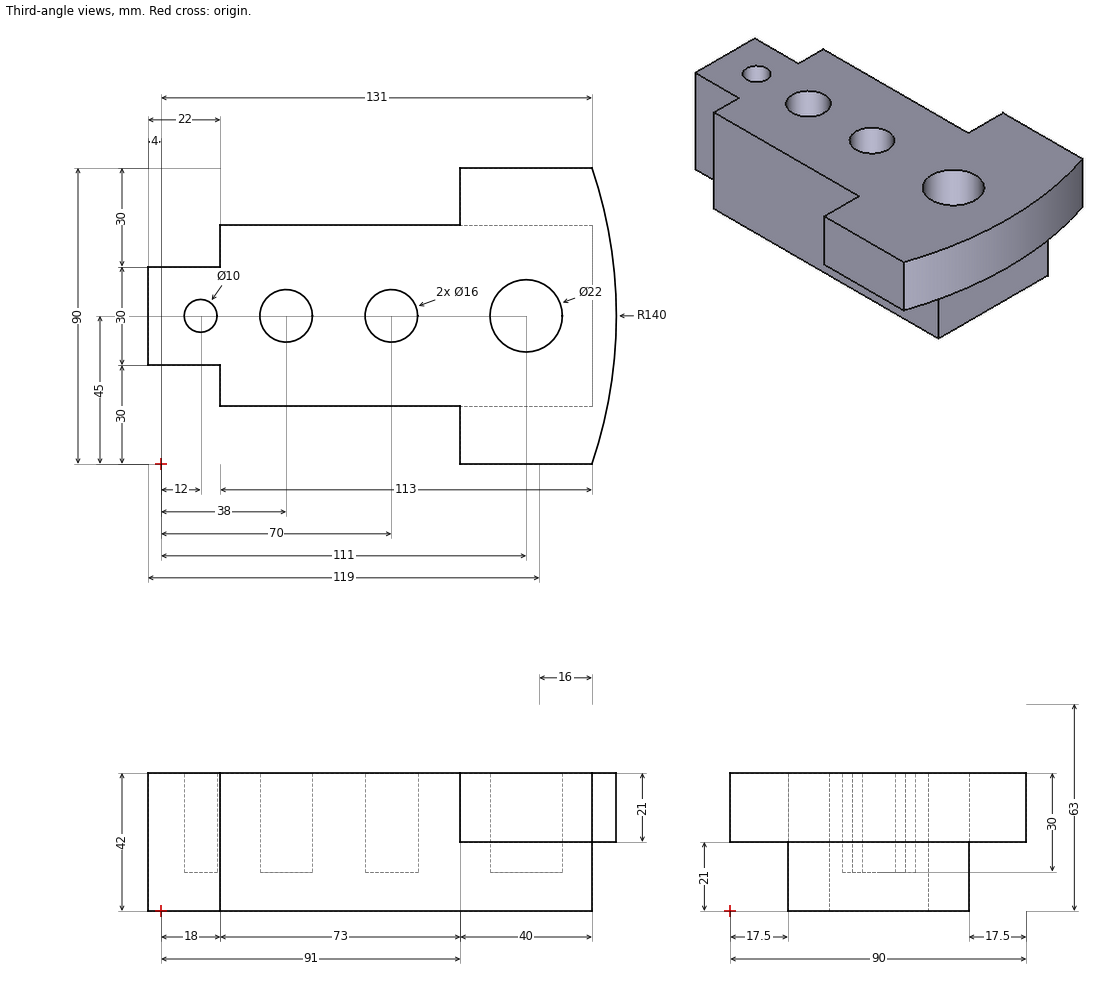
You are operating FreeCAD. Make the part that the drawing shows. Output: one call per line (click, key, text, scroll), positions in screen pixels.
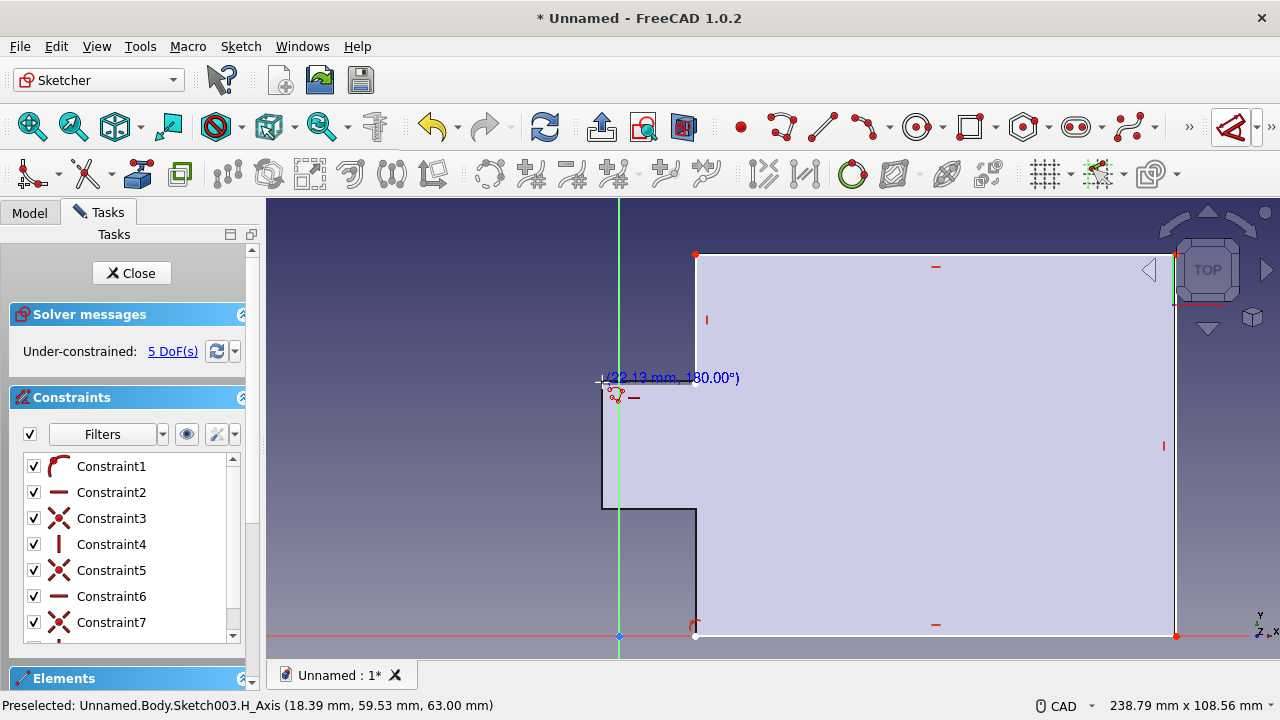
click(602, 382)
click(602, 509)
click(696, 509)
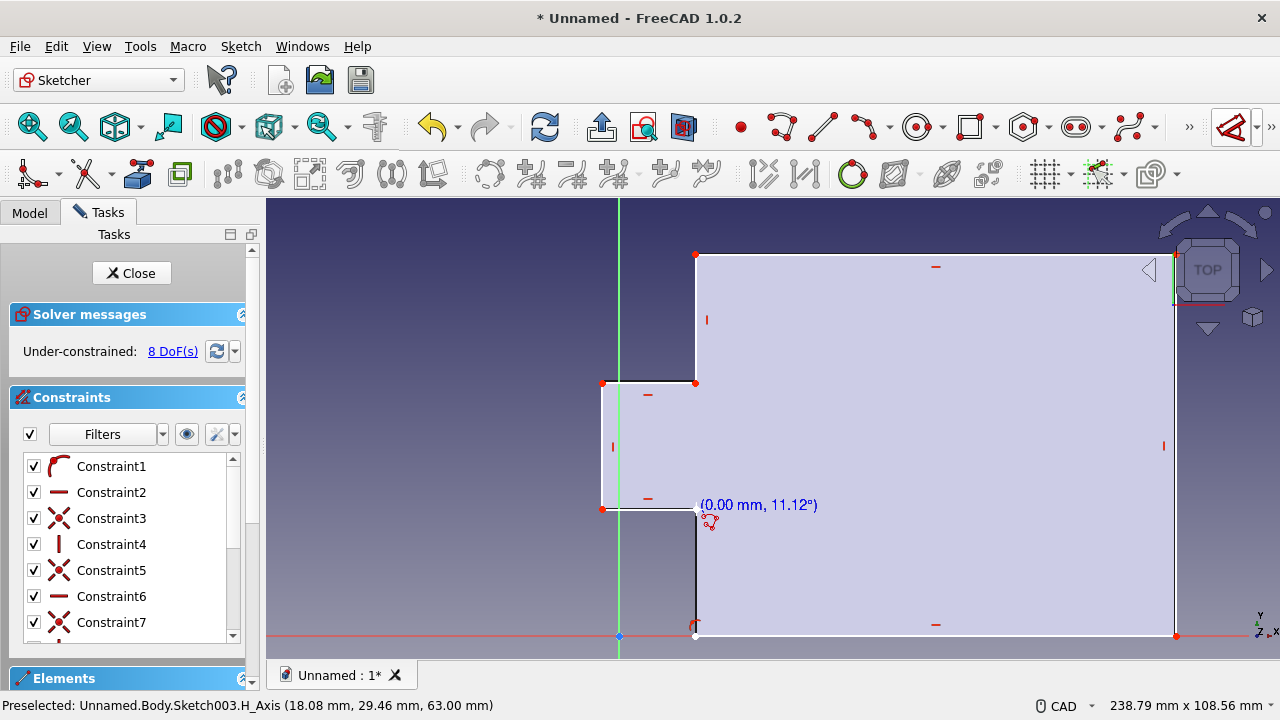
scroll(294, 354, down, 1)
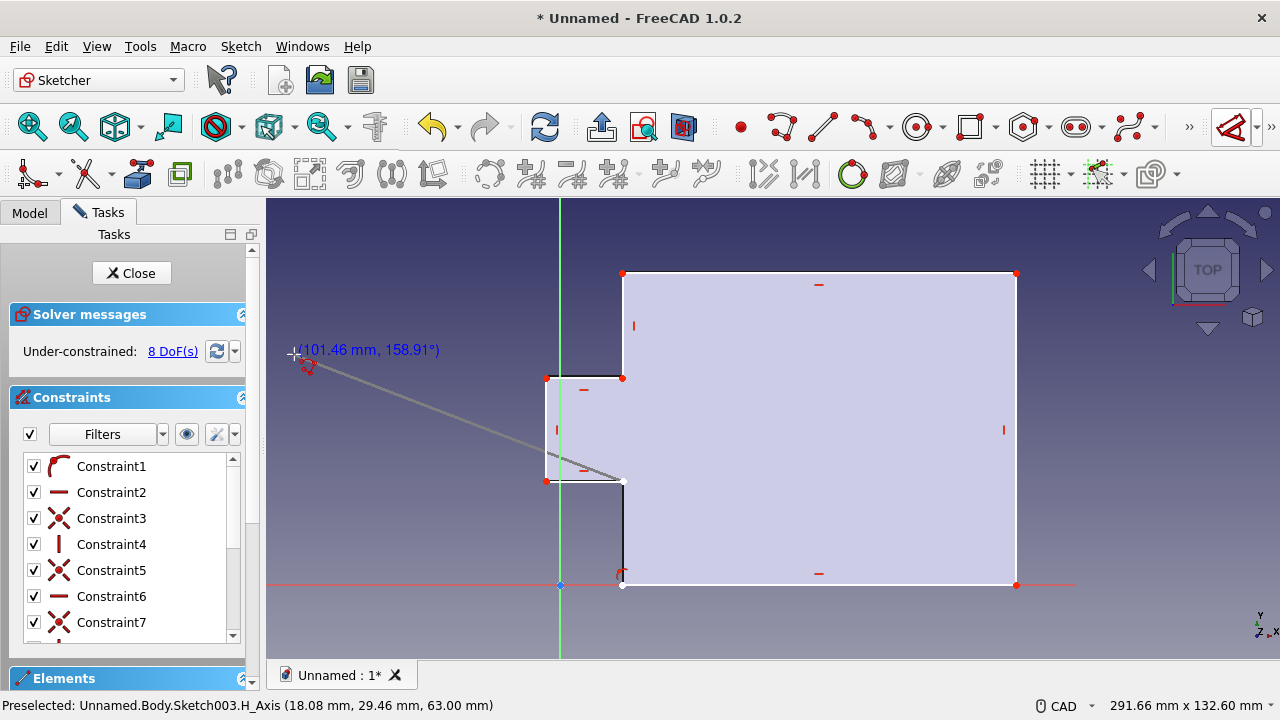
click(623, 585)
key(Escape)
key(Escape)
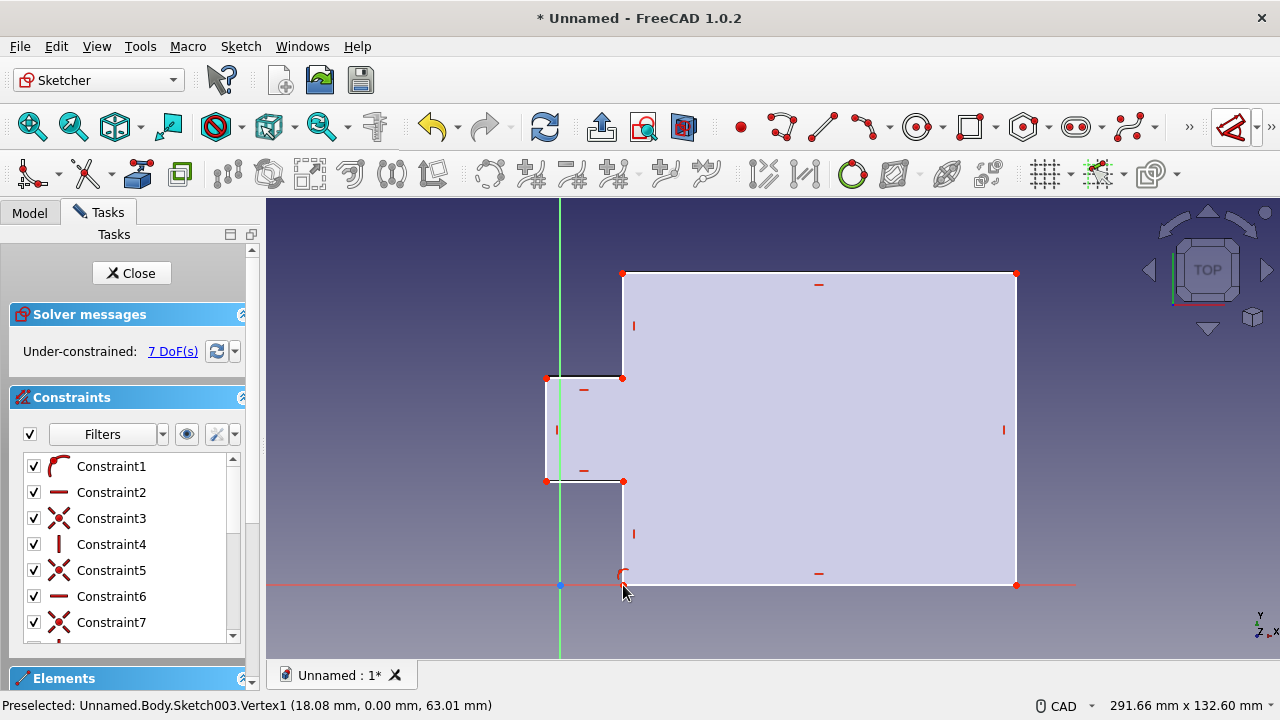
click(1016, 491)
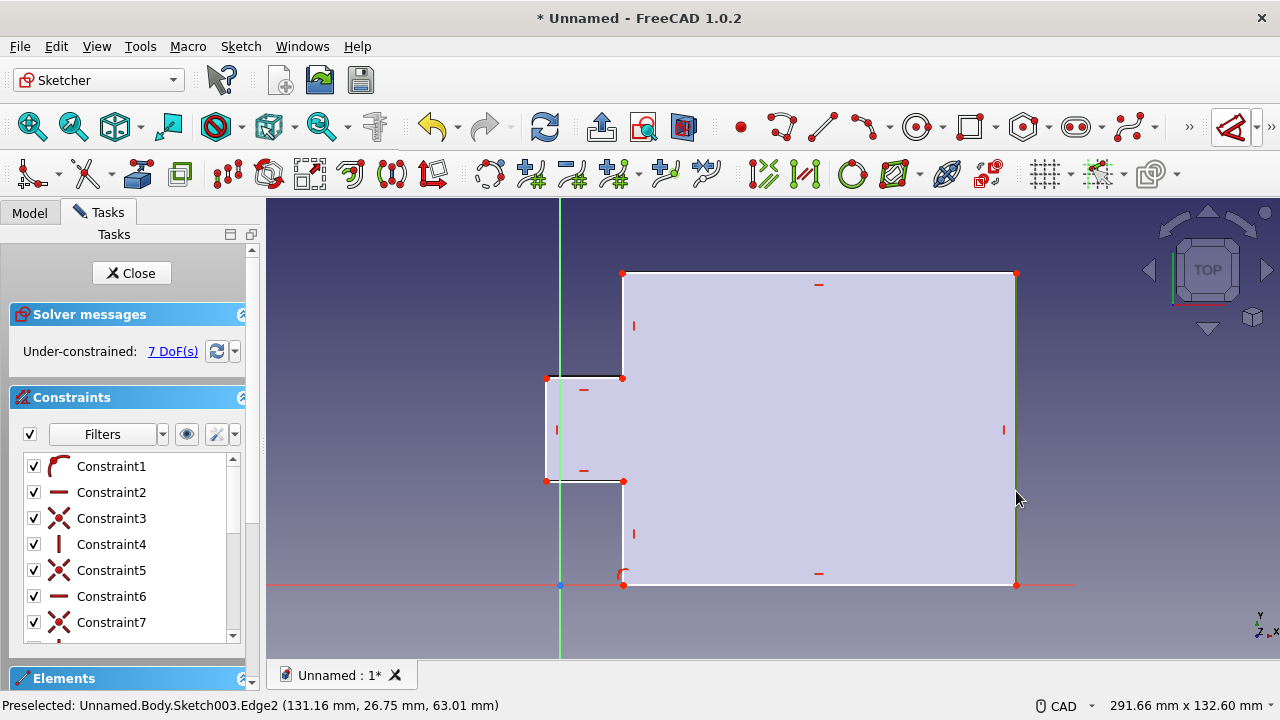
key(i)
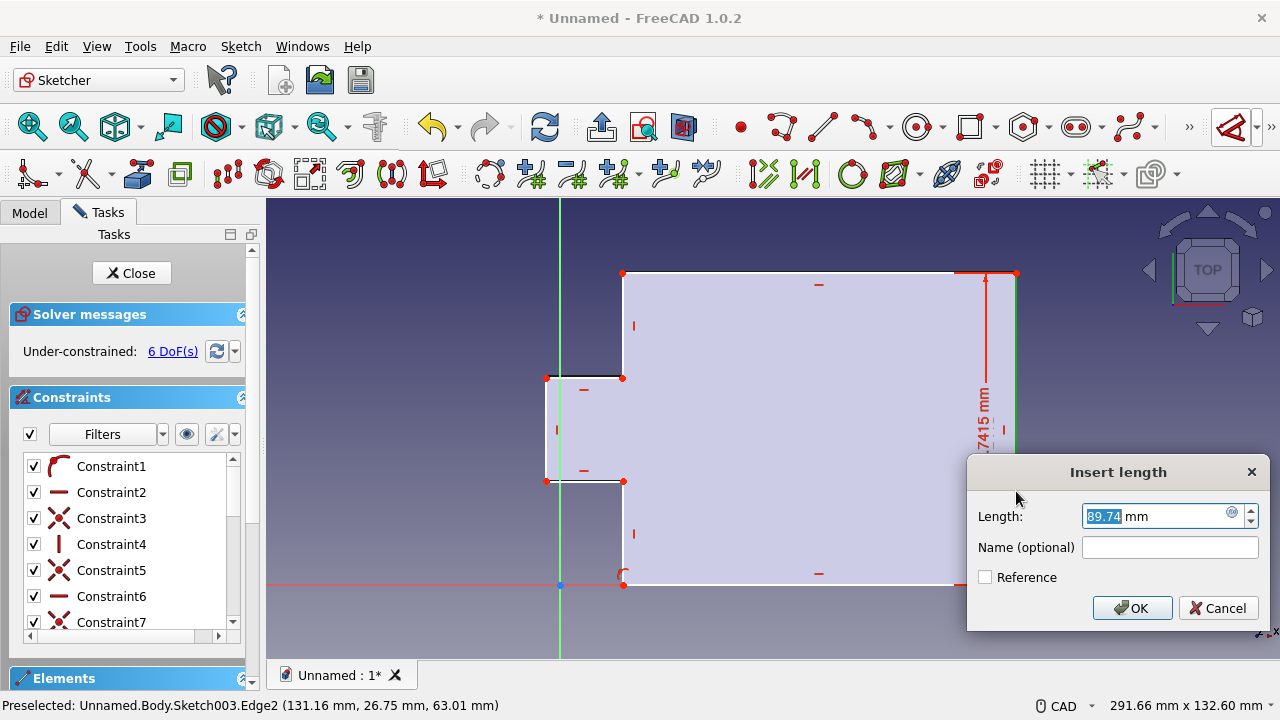
text(90)
key(Return)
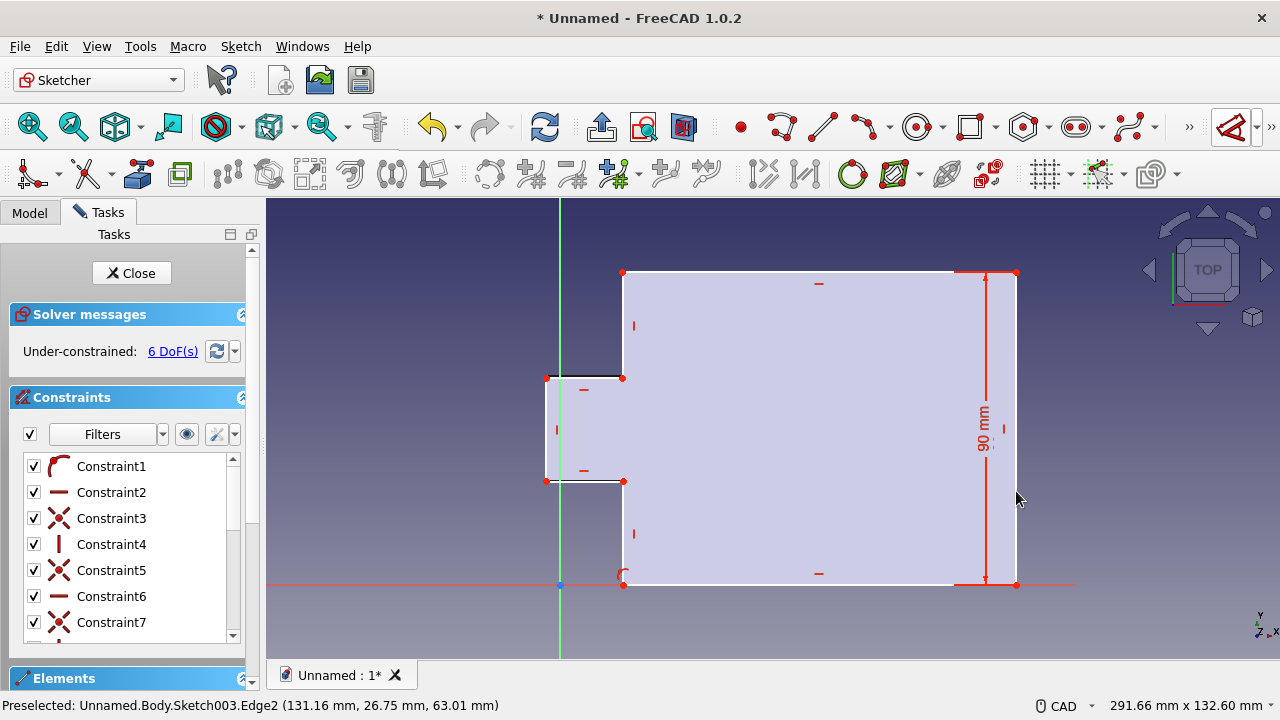
click(623, 304)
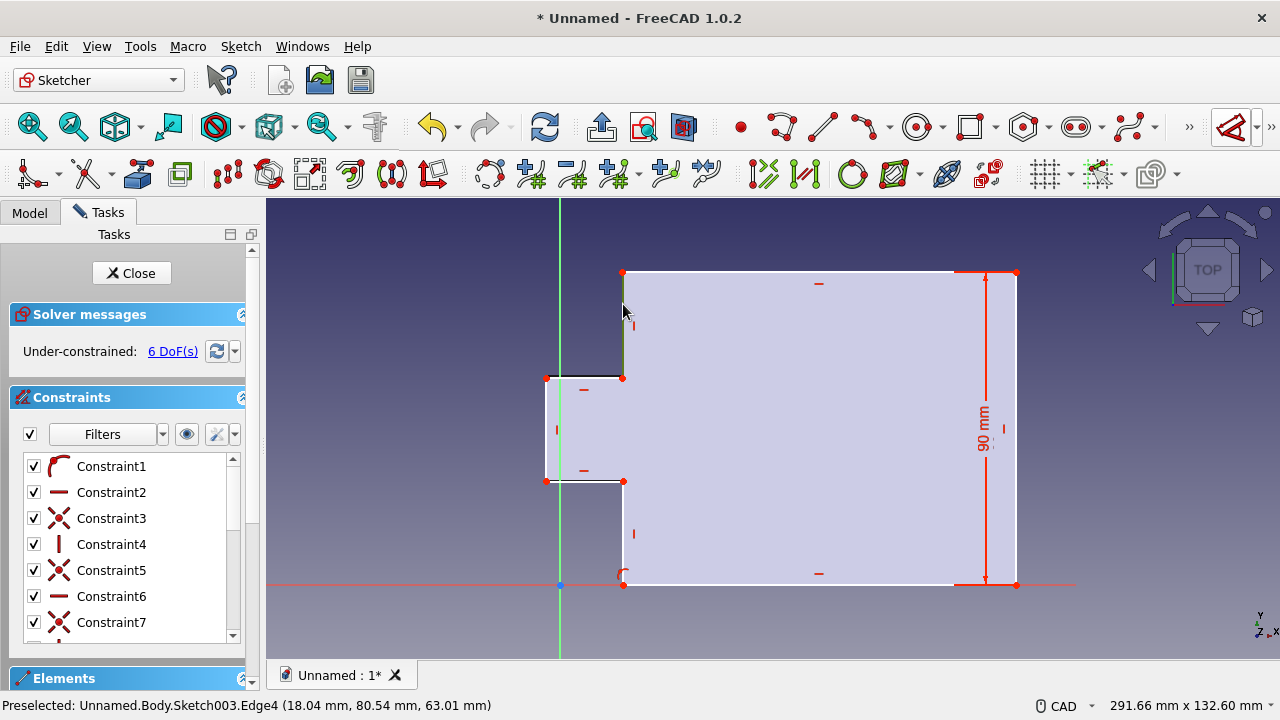
click(1256, 128)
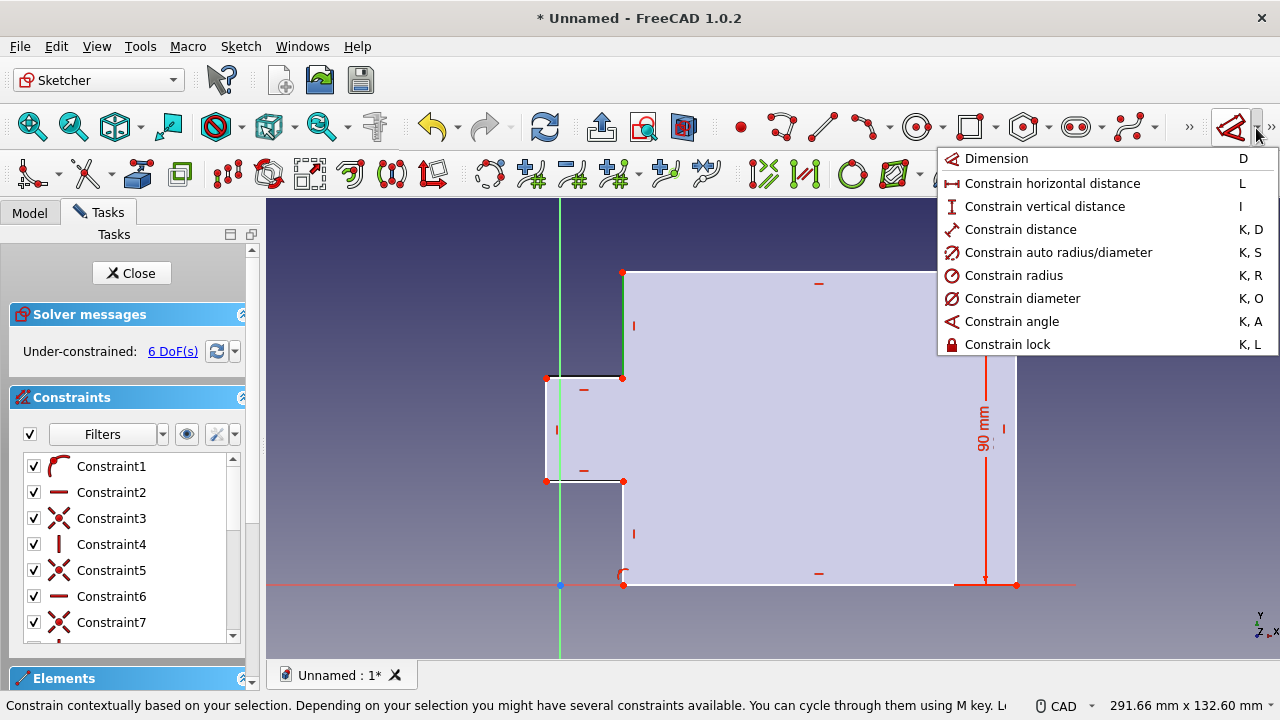
click(1108, 206)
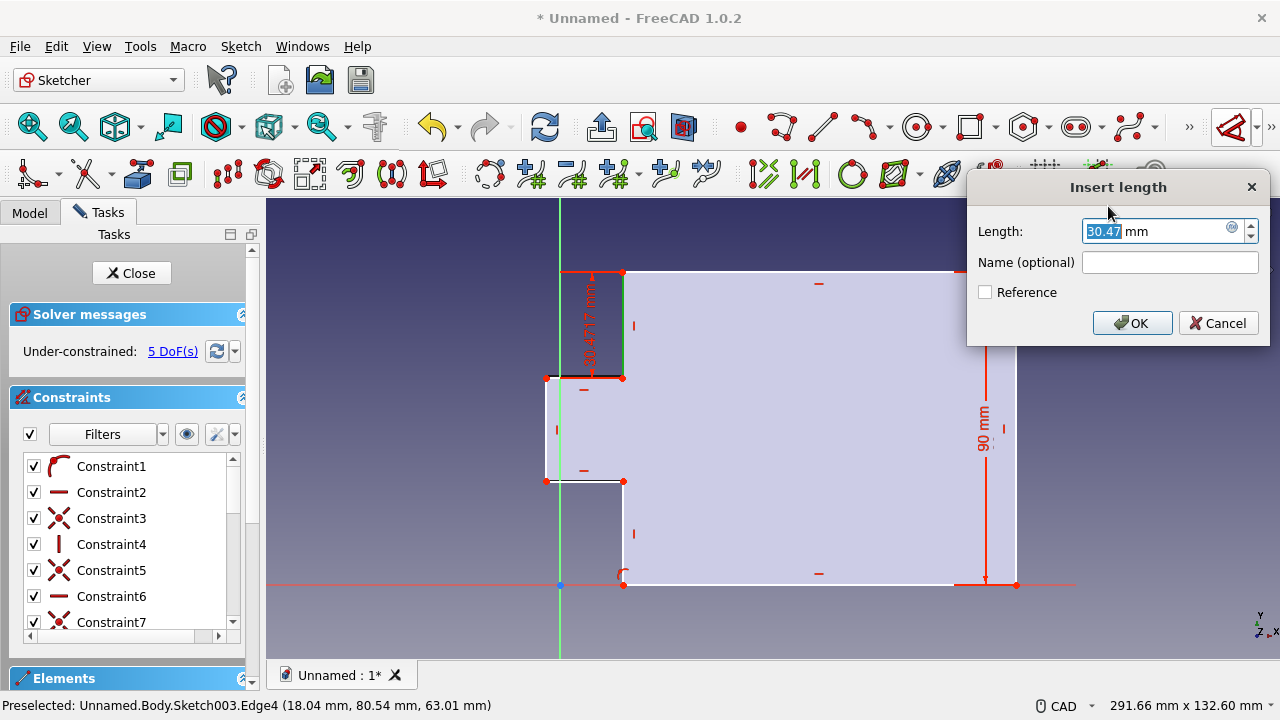
text(30)
key(Return)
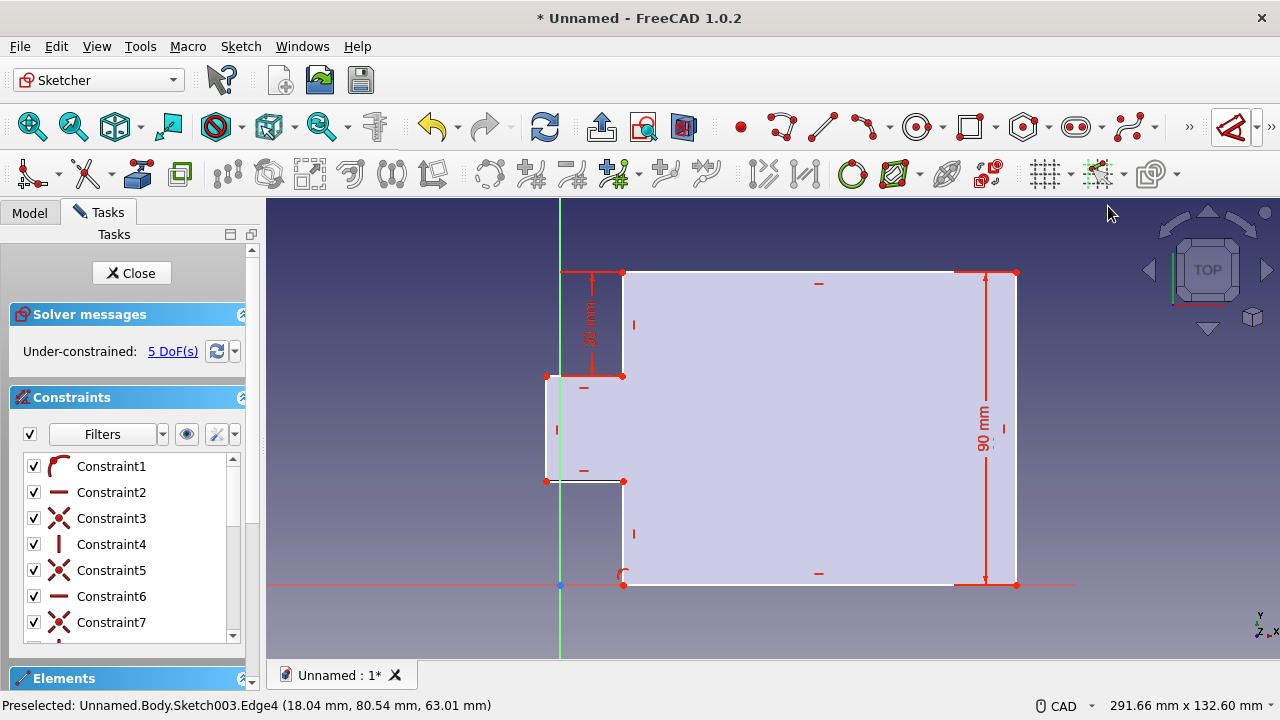
click(600, 376)